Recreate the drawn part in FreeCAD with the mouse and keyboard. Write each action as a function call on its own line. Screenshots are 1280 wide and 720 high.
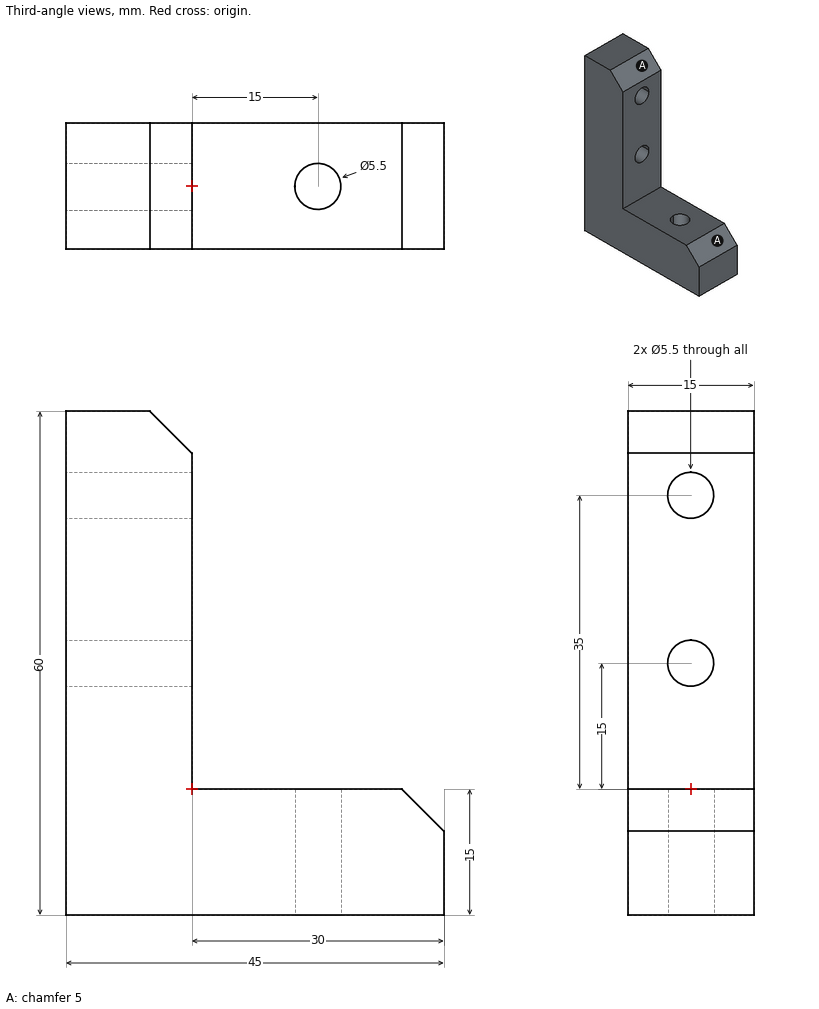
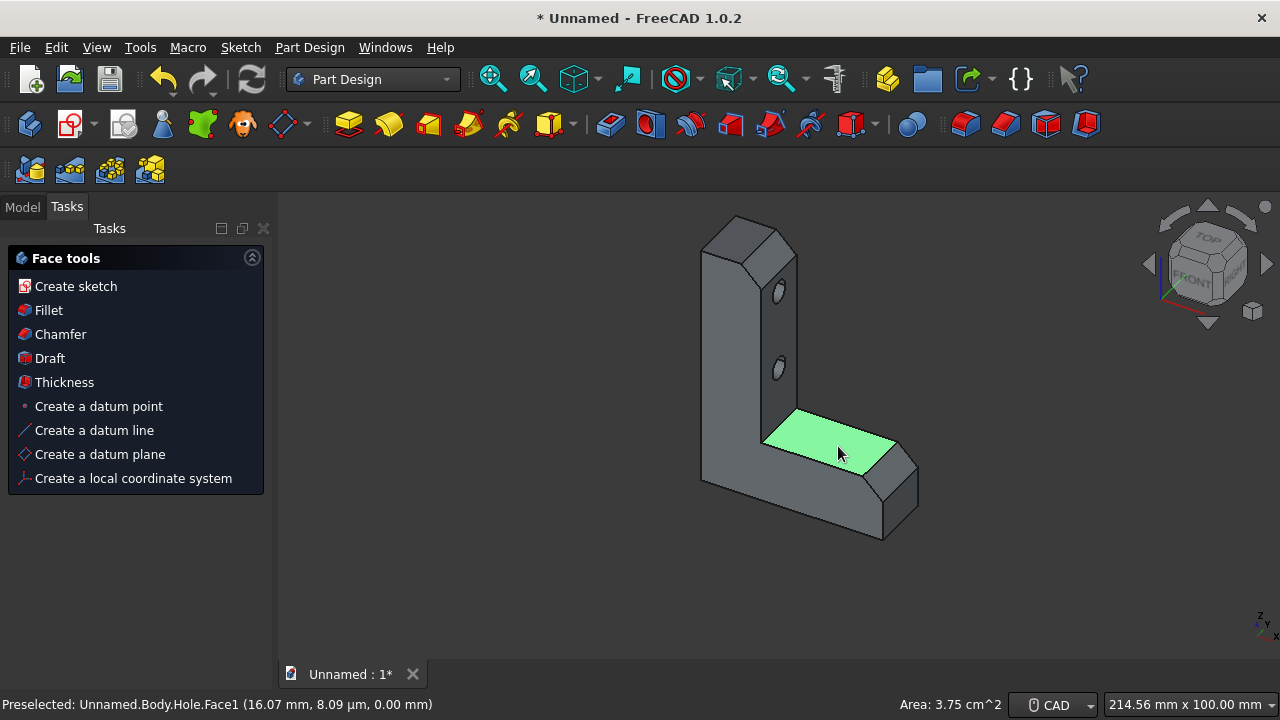
click(70, 124)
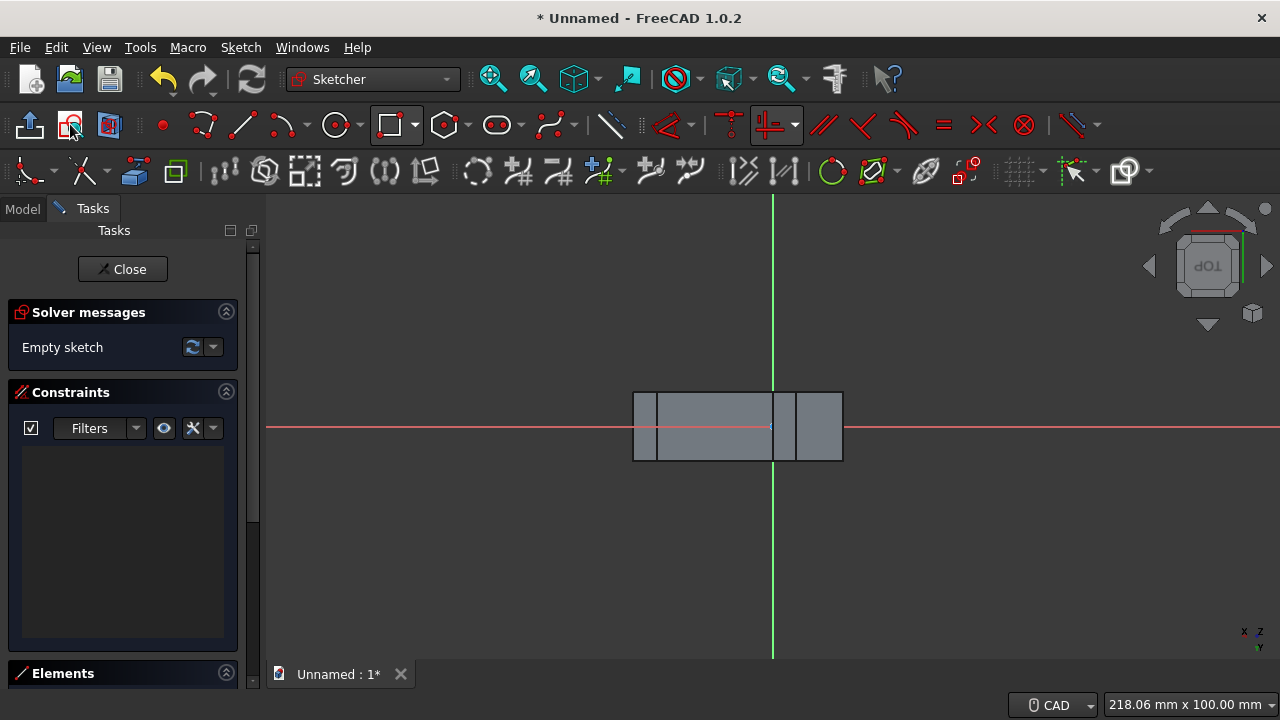
scroll(703, 426, up, 12)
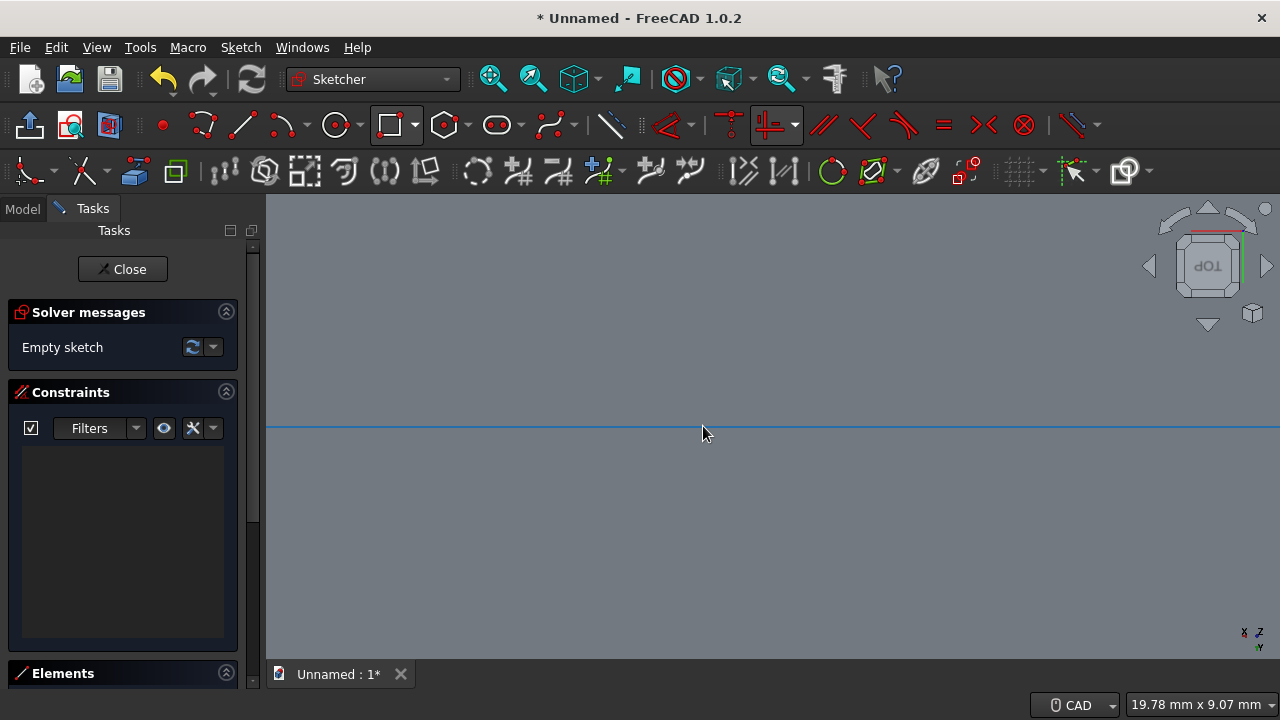
click(336, 126)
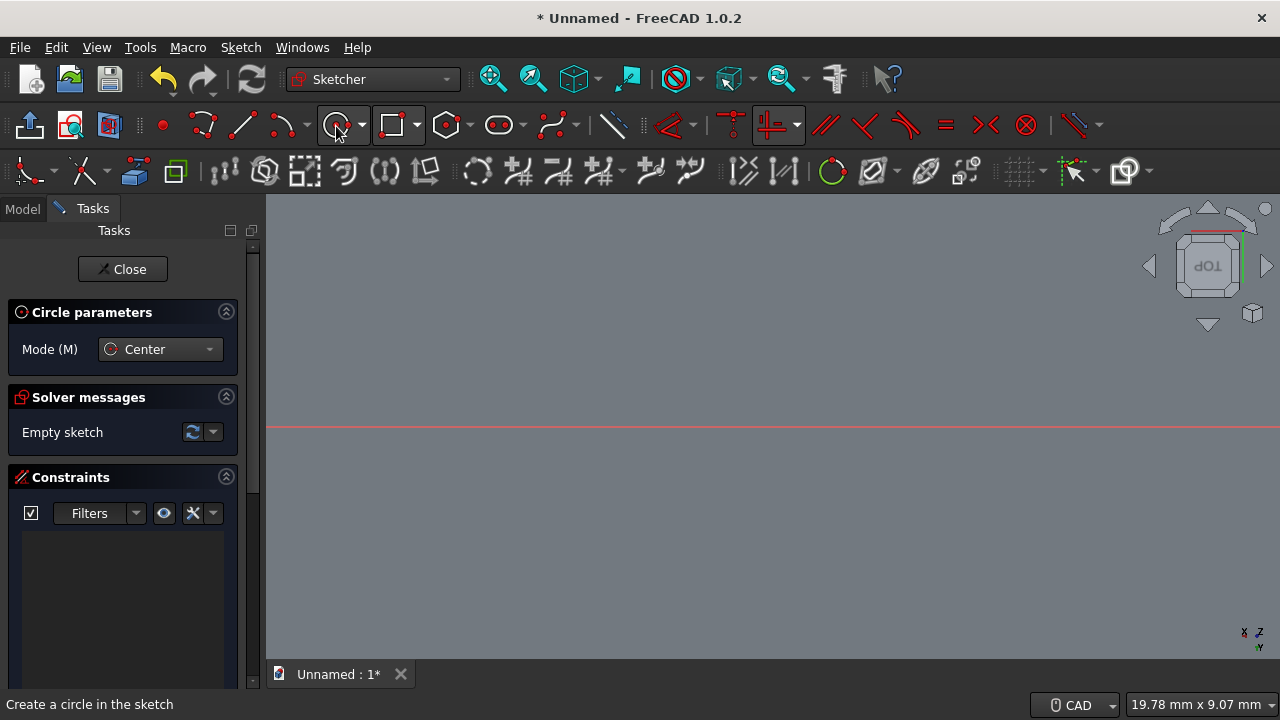
click(701, 426)
move(801, 327)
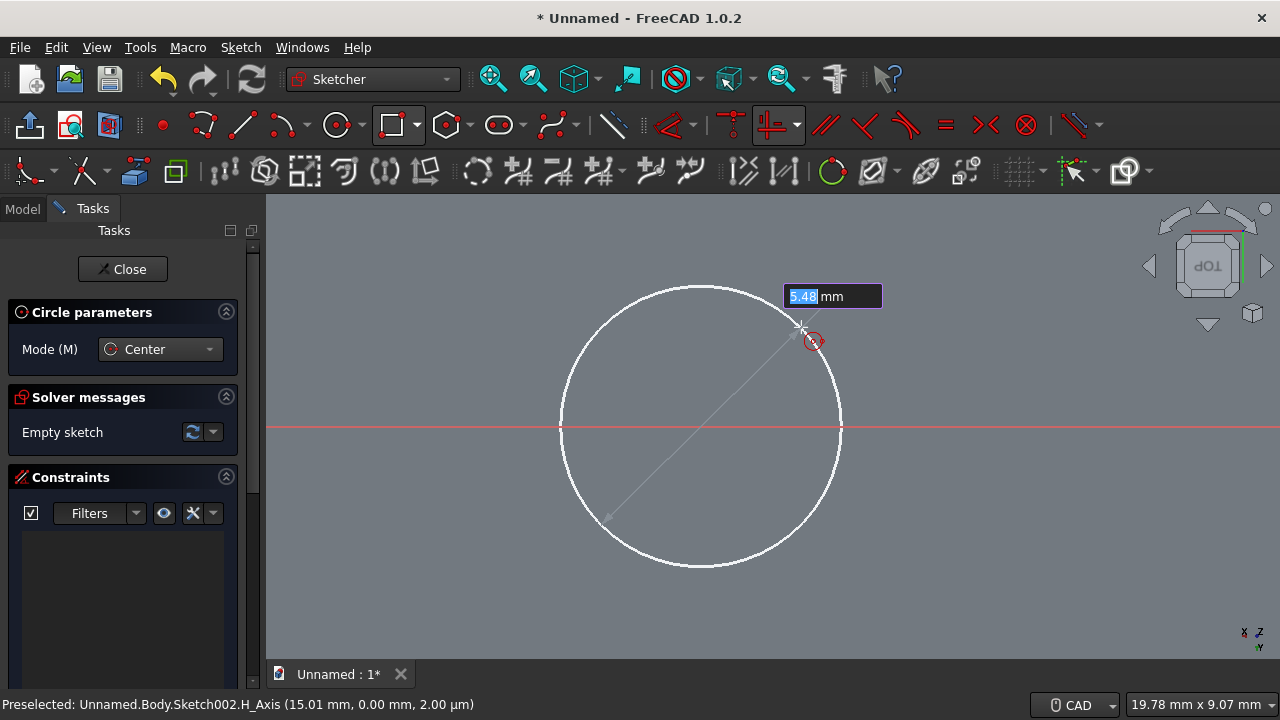
text(5.5)
key(Return)
key(Escape)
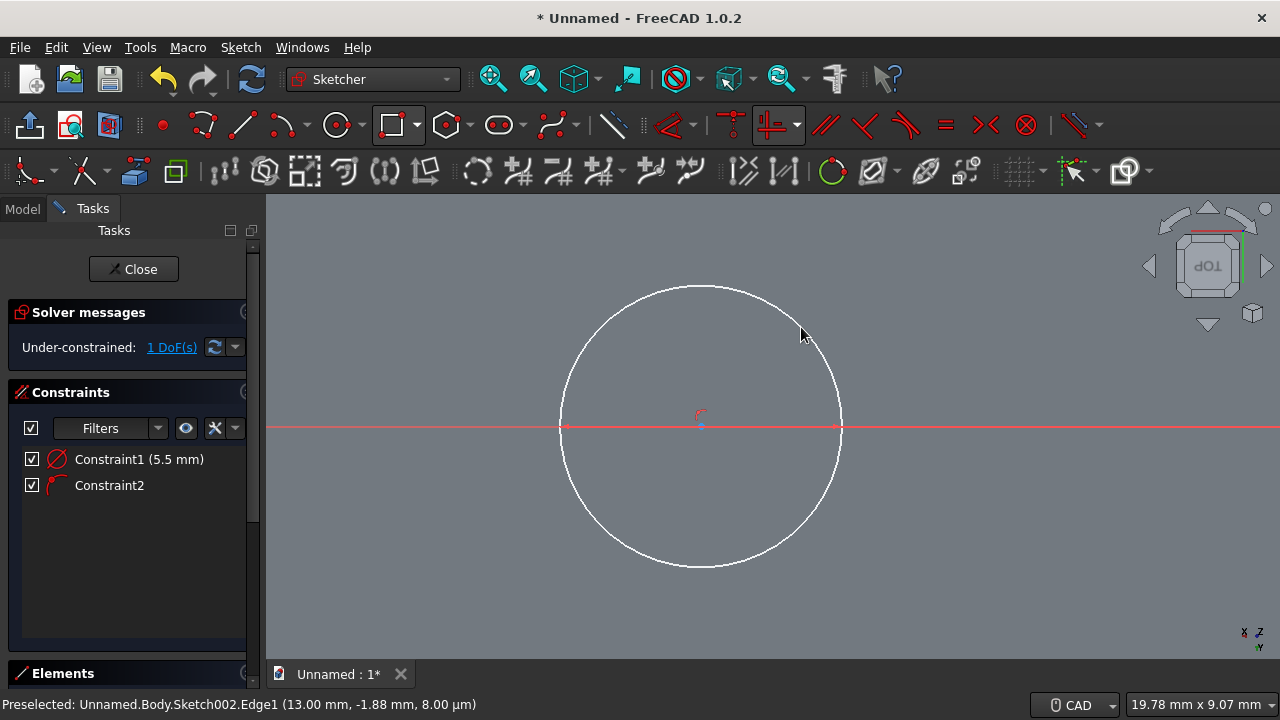
key(d)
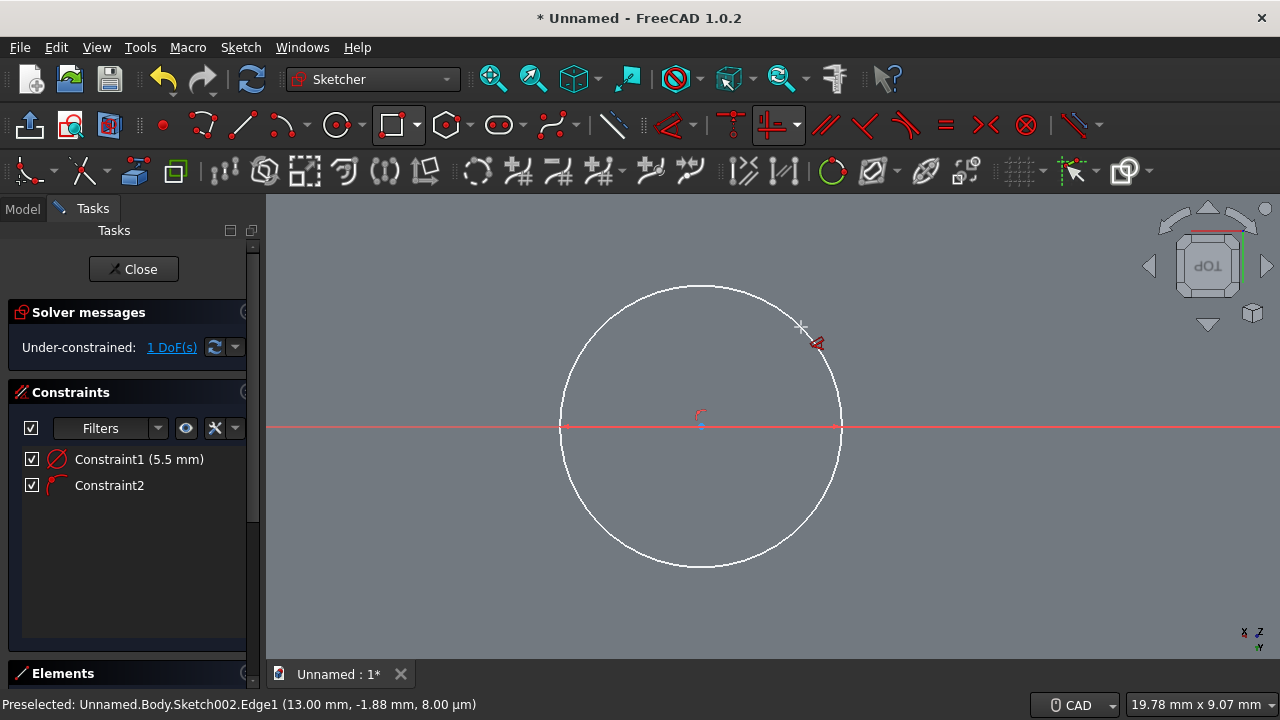
click(701, 426)
click(908, 460)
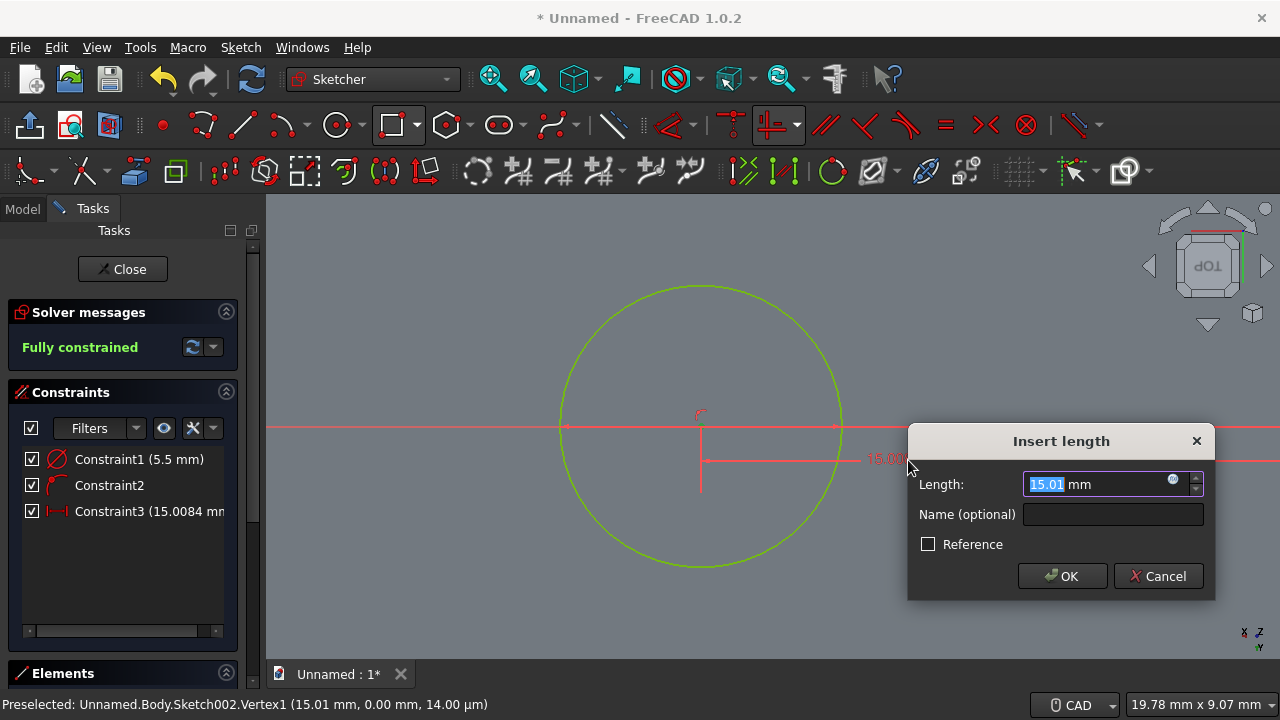
text(15)
key(Return)
key(Escape)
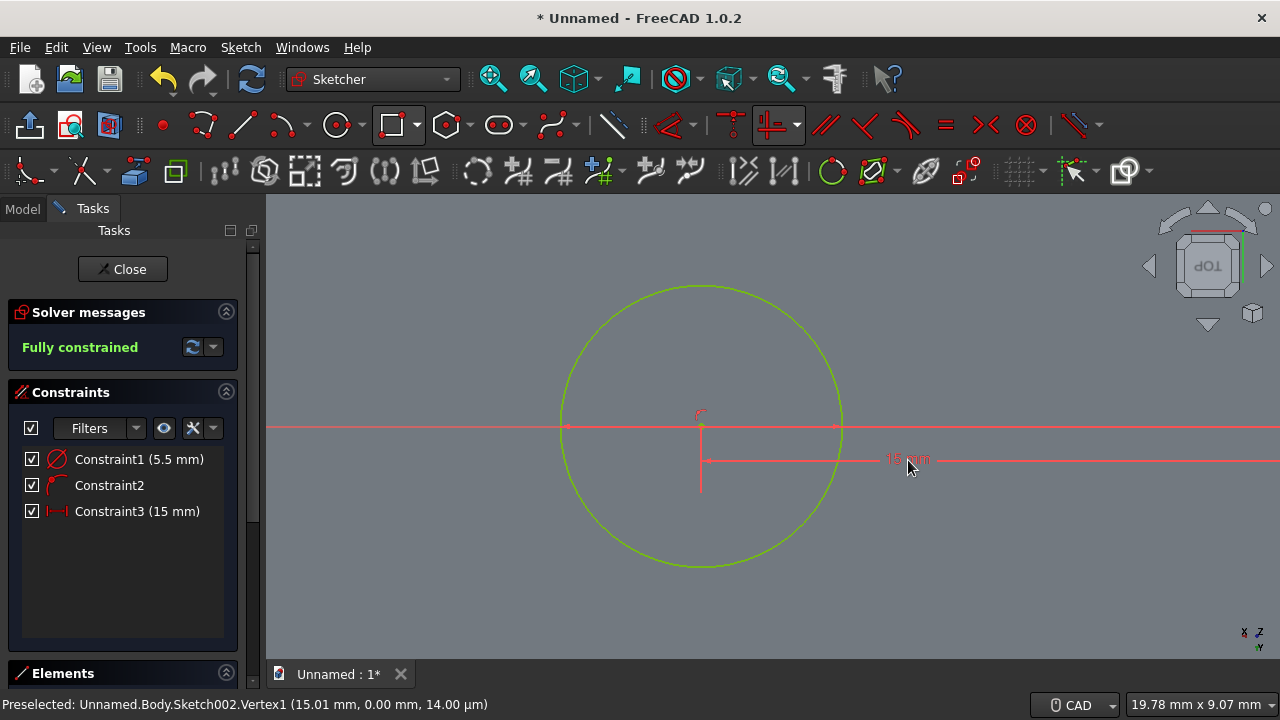
click(123, 269)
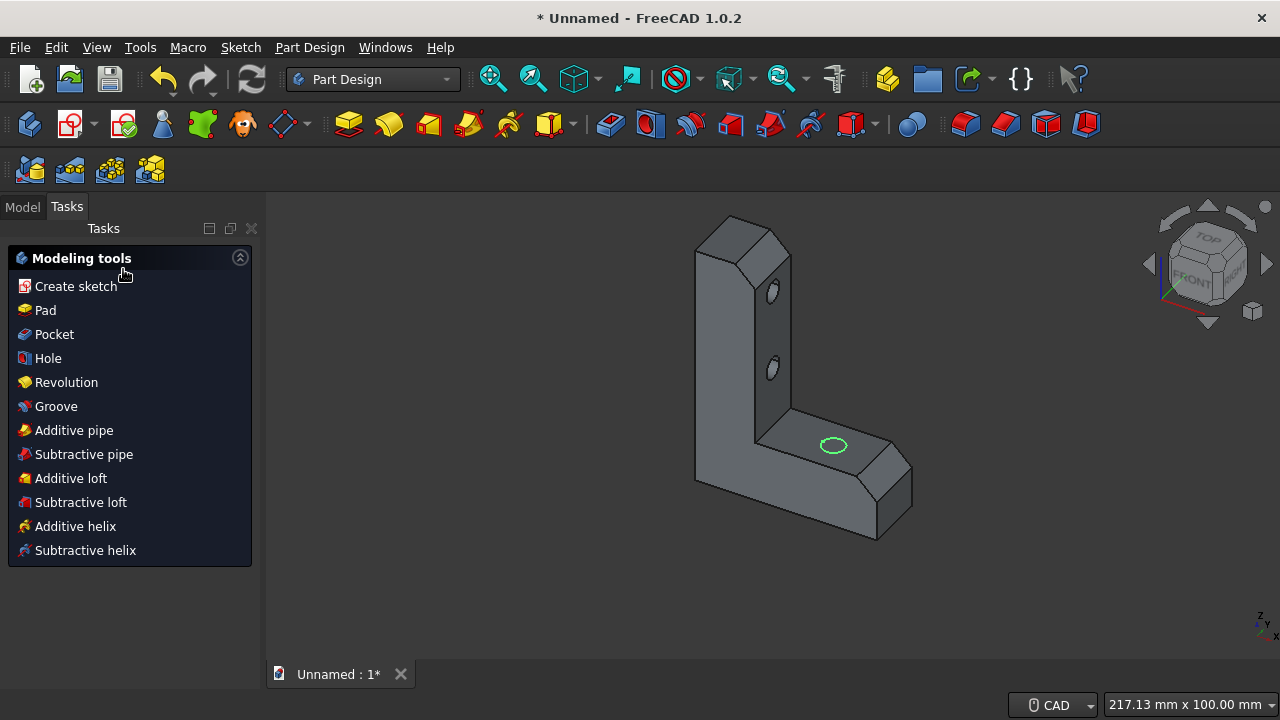
click(612, 124)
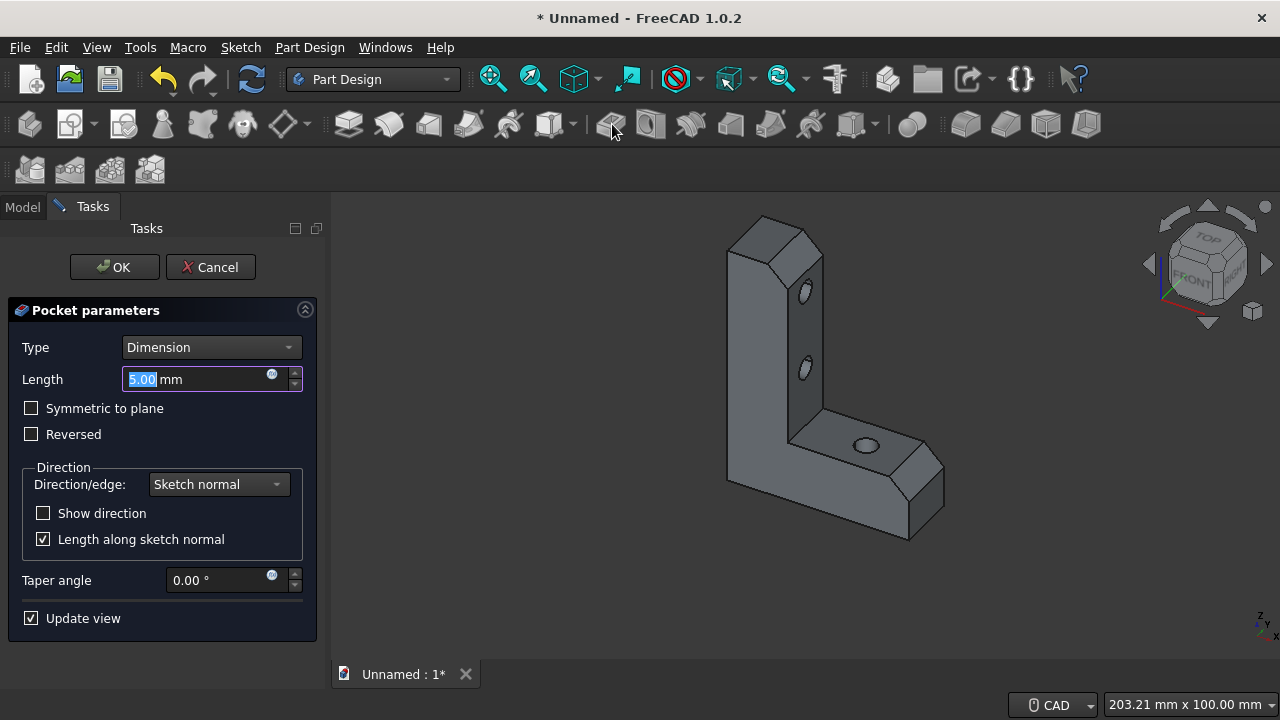
click(212, 348)